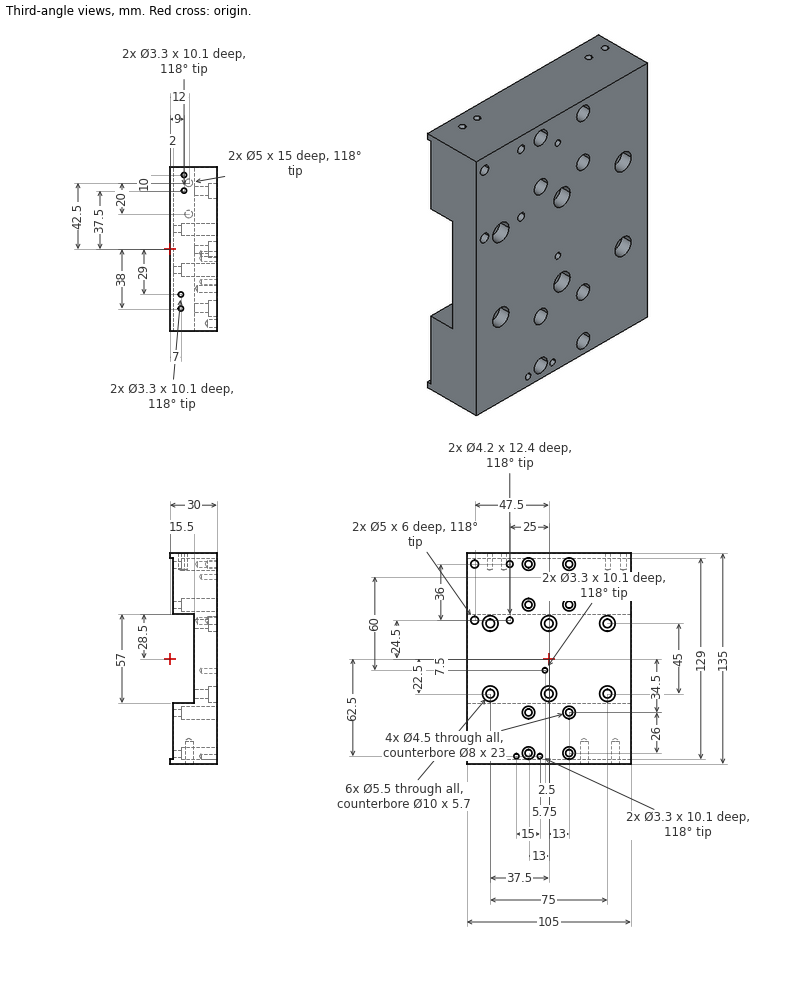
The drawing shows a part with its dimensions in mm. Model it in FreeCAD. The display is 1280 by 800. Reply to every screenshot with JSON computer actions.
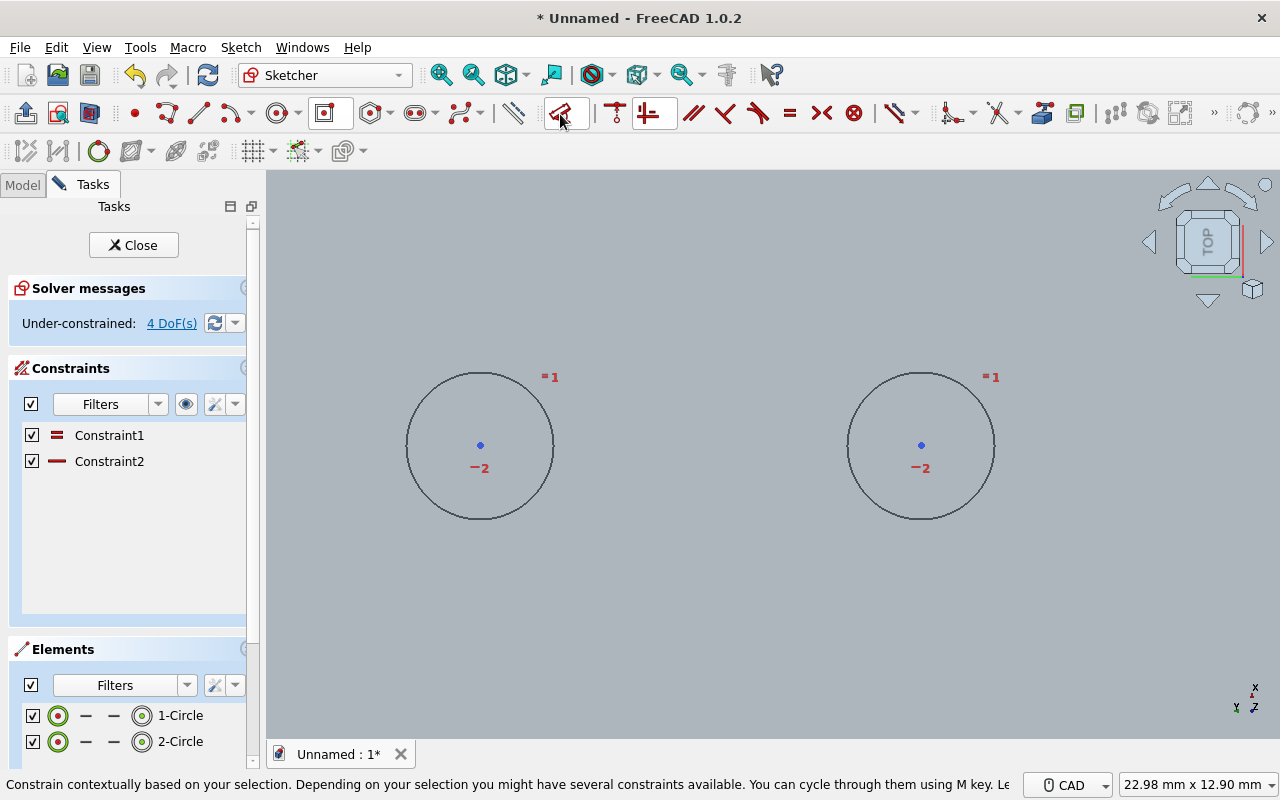
{"action": "left_click", "coordinate": [973, 394]}
{"action": "left_click", "coordinate": [996, 371]}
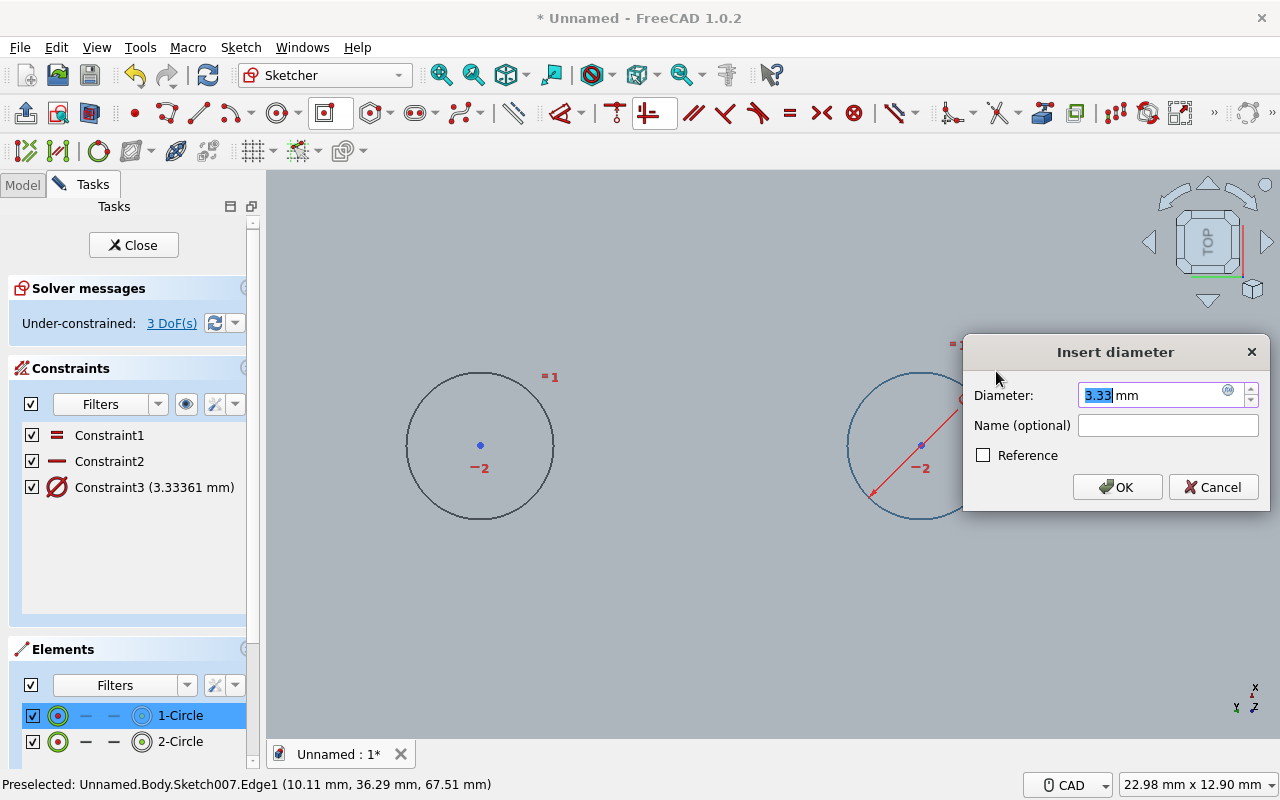
{"action": "type", "text": "3.3"}
{"action": "key", "text": "Return"}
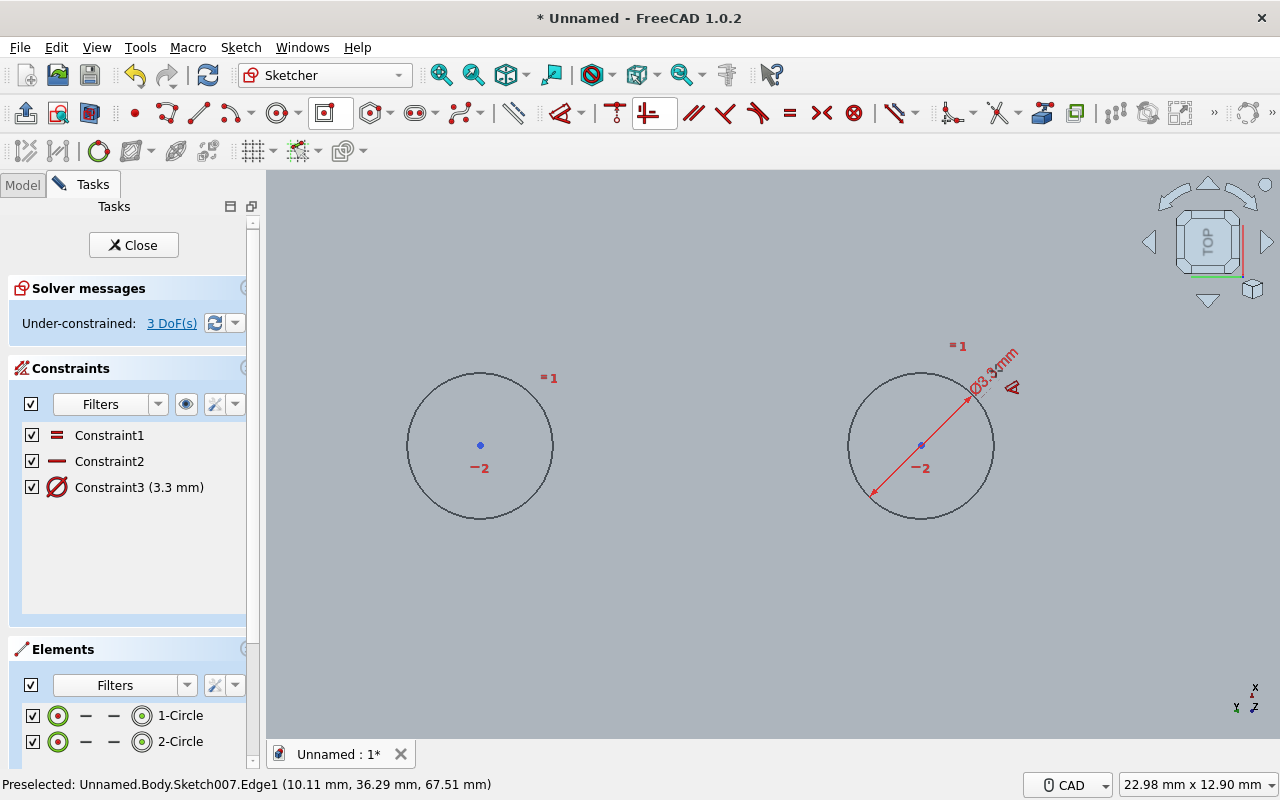
{"action": "left_click", "coordinate": [921, 446]}
{"action": "left_click", "coordinate": [887, 579]}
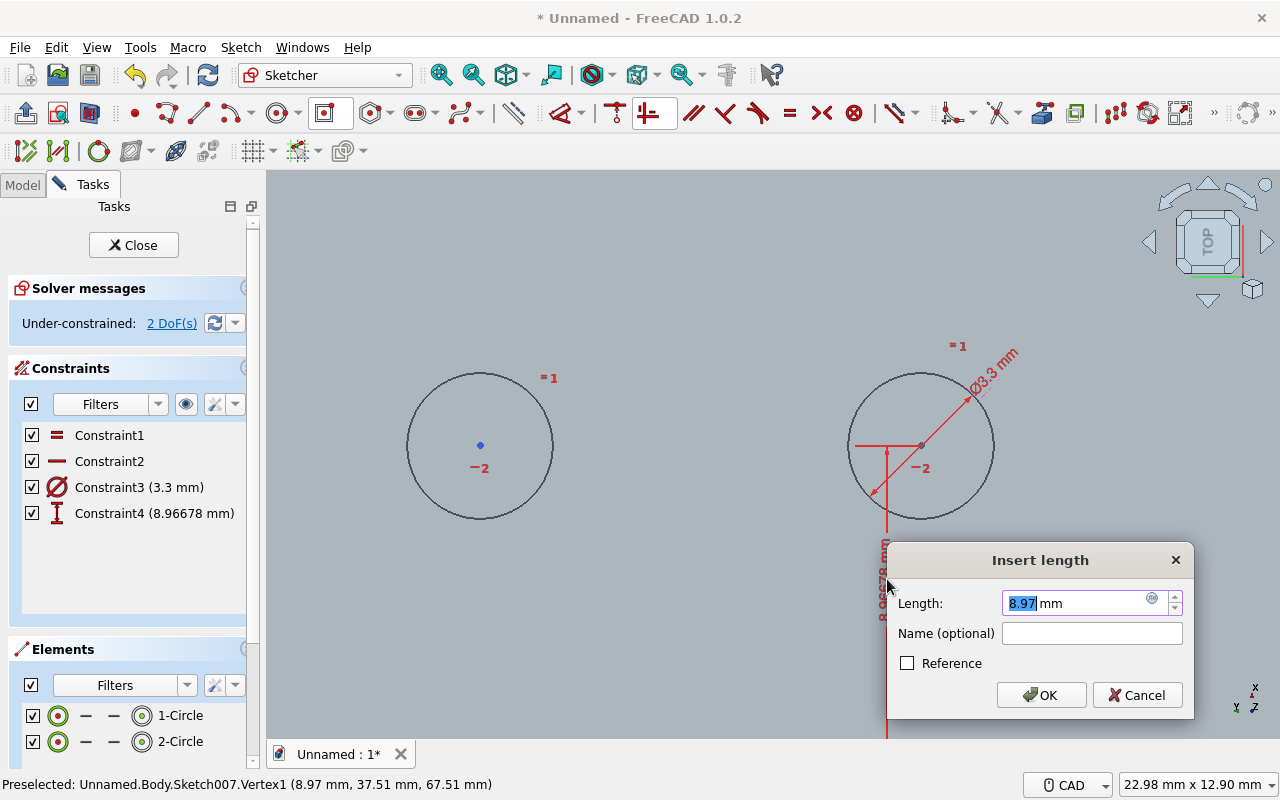
{"action": "type", "text": "9"}
{"action": "key", "text": "Return"}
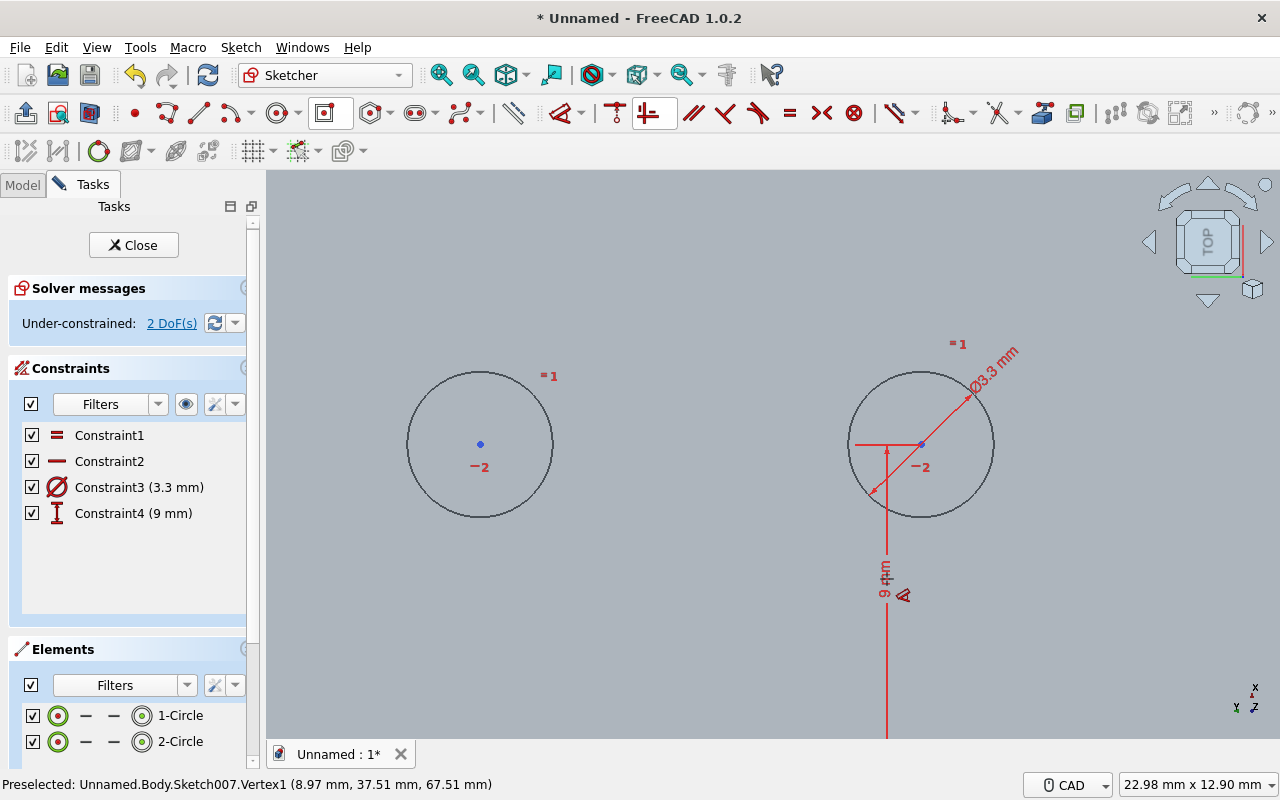
{"action": "left_click", "coordinate": [921, 445]}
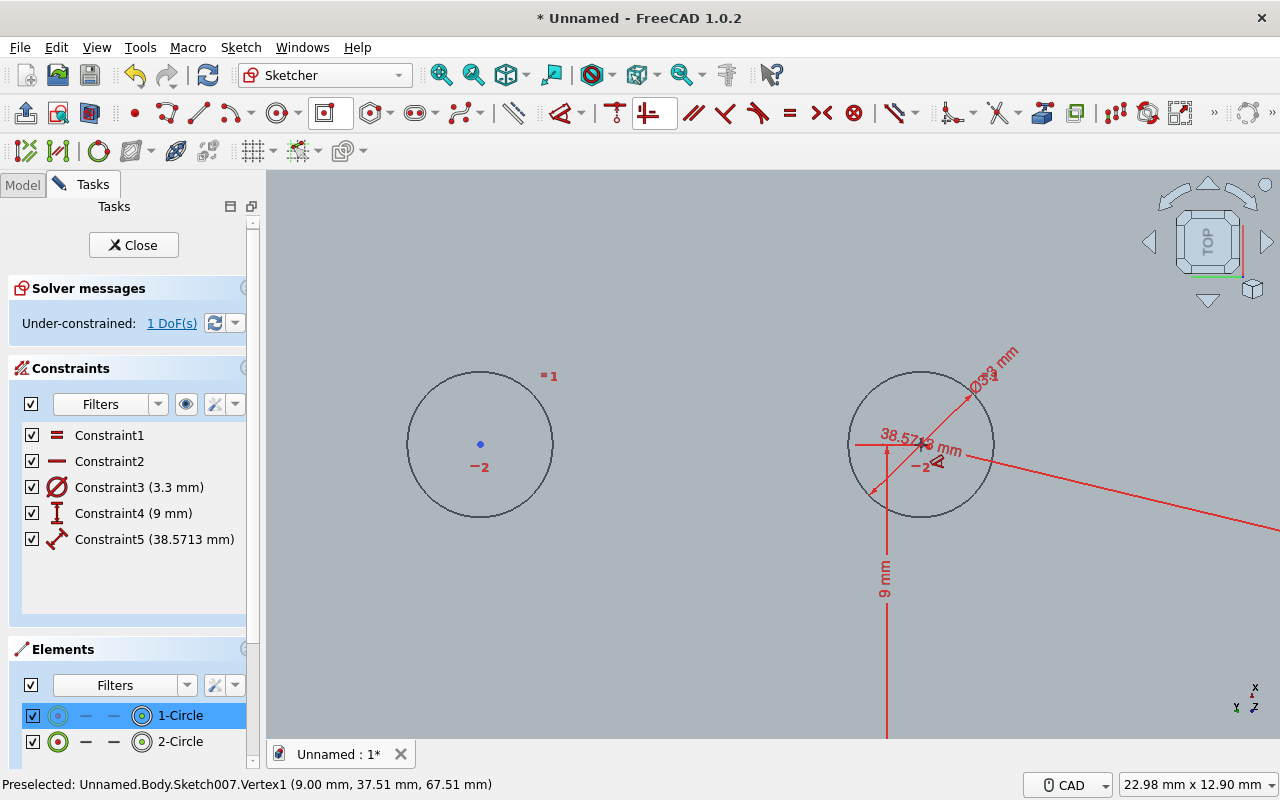
{"action": "left_click", "coordinate": [480, 445]}
{"action": "left_click", "coordinate": [701, 411]}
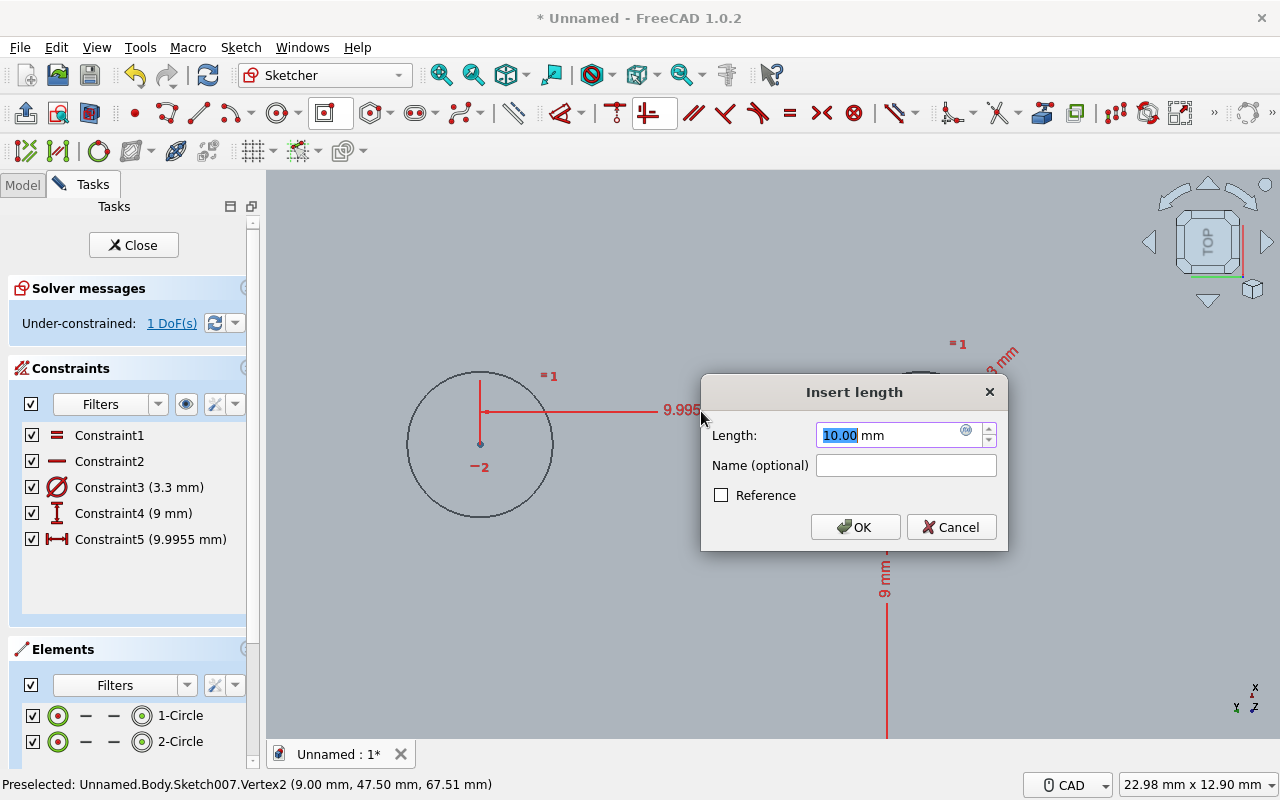
{"action": "type", "text": "10"}
{"action": "key", "text": "Return"}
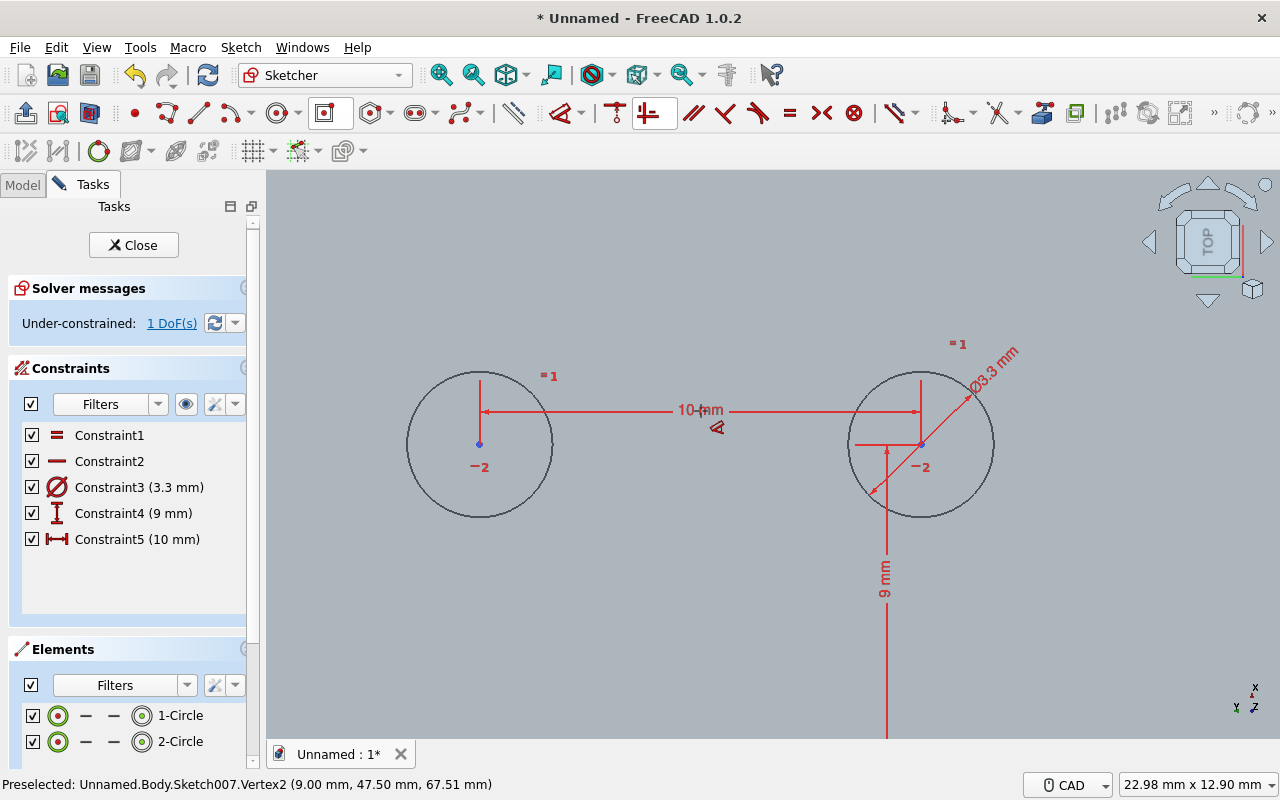
{"action": "left_click", "coordinate": [921, 445]}
{"action": "left_click", "coordinate": [1018, 411]}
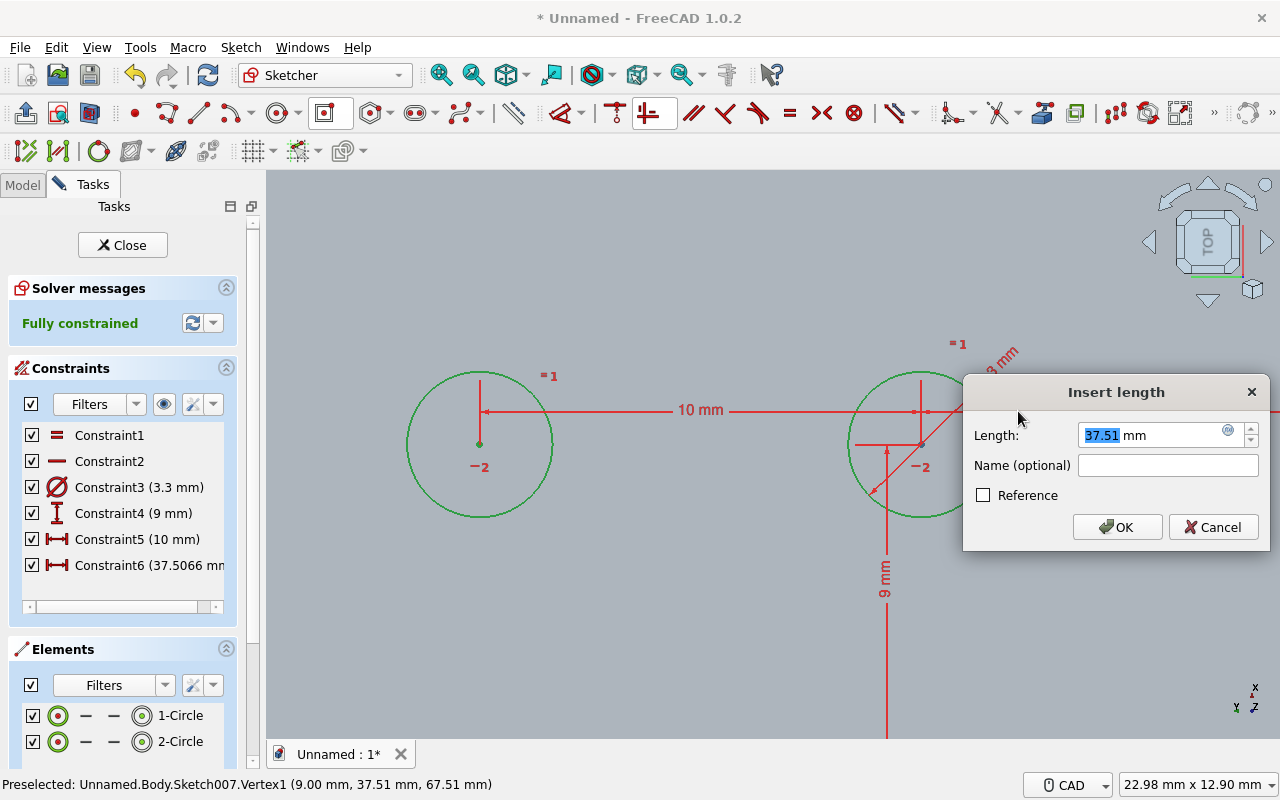
{"action": "type", "text": "37.5"}
{"action": "key", "text": "Return"}
{"action": "key", "text": "Escape"}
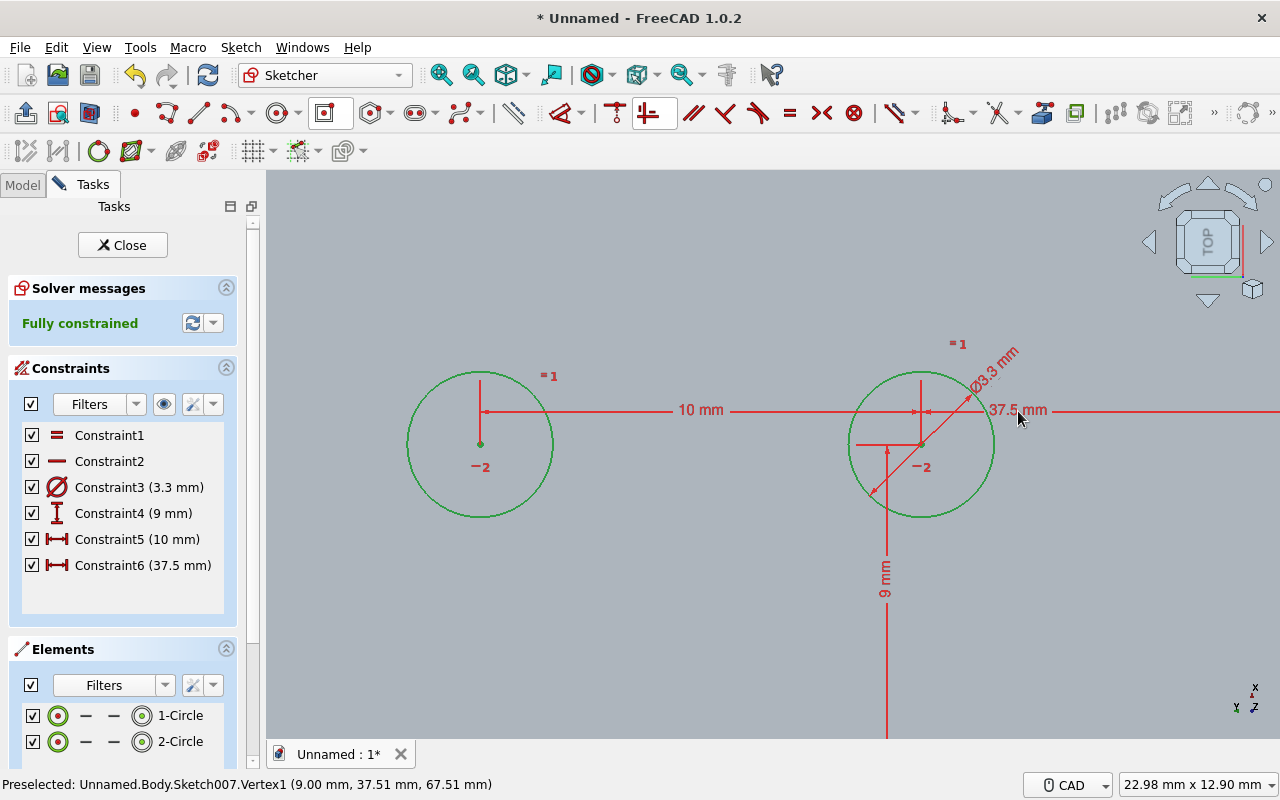
{"action": "left_click", "coordinate": [123, 245]}